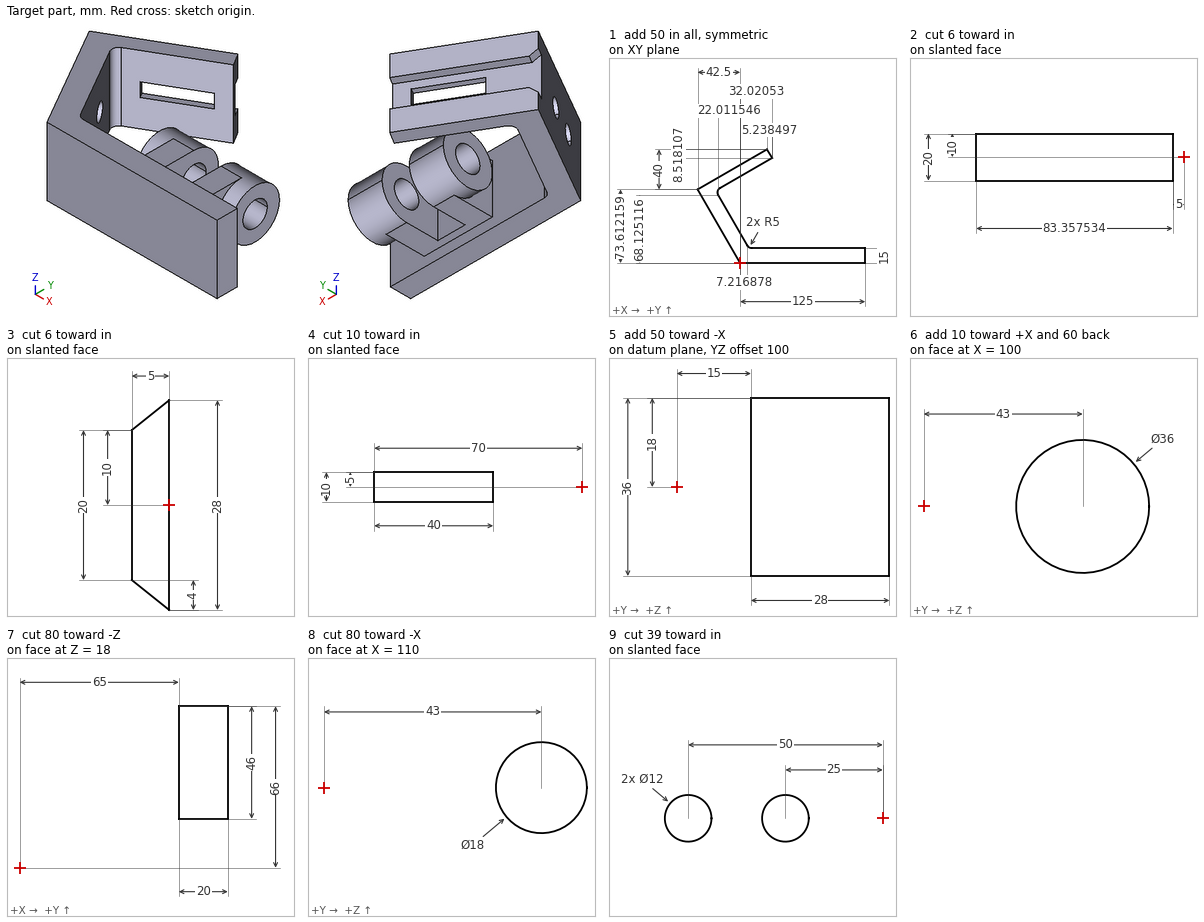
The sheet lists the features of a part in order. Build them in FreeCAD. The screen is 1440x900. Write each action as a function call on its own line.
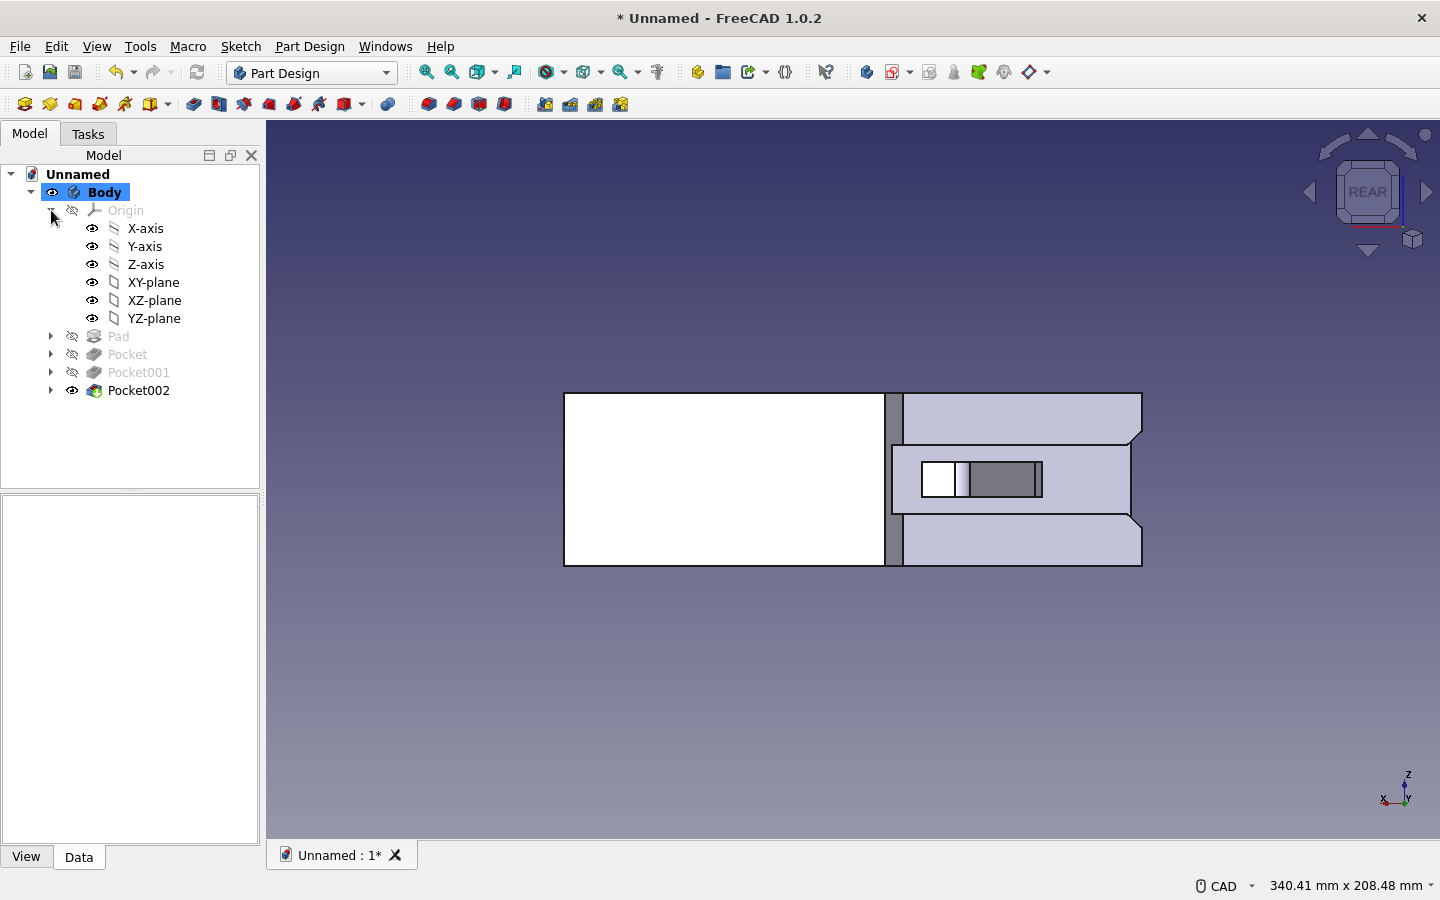
click(137, 318)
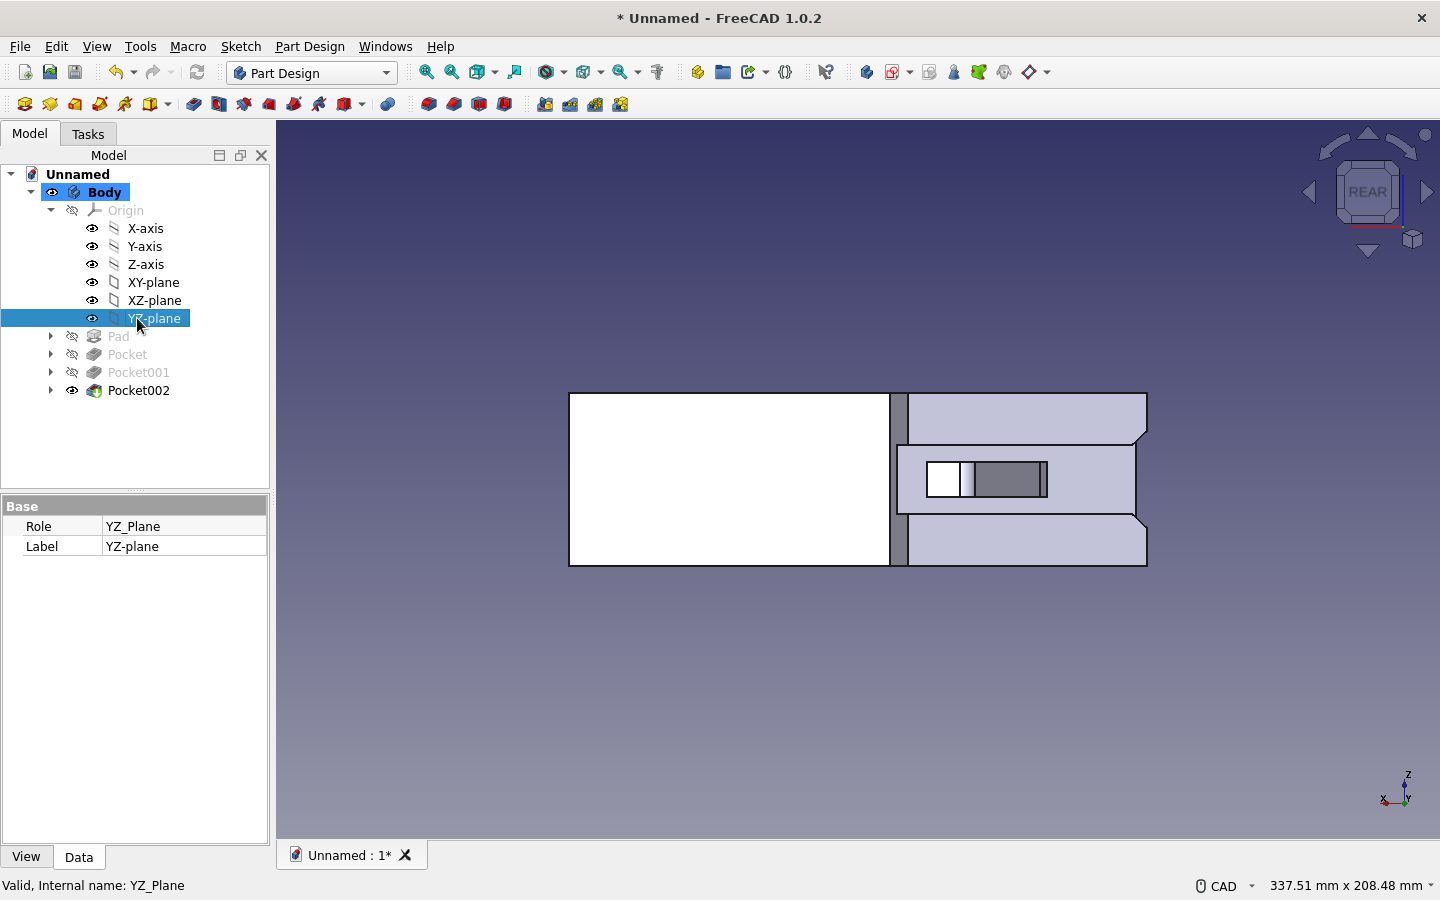
click(1028, 72)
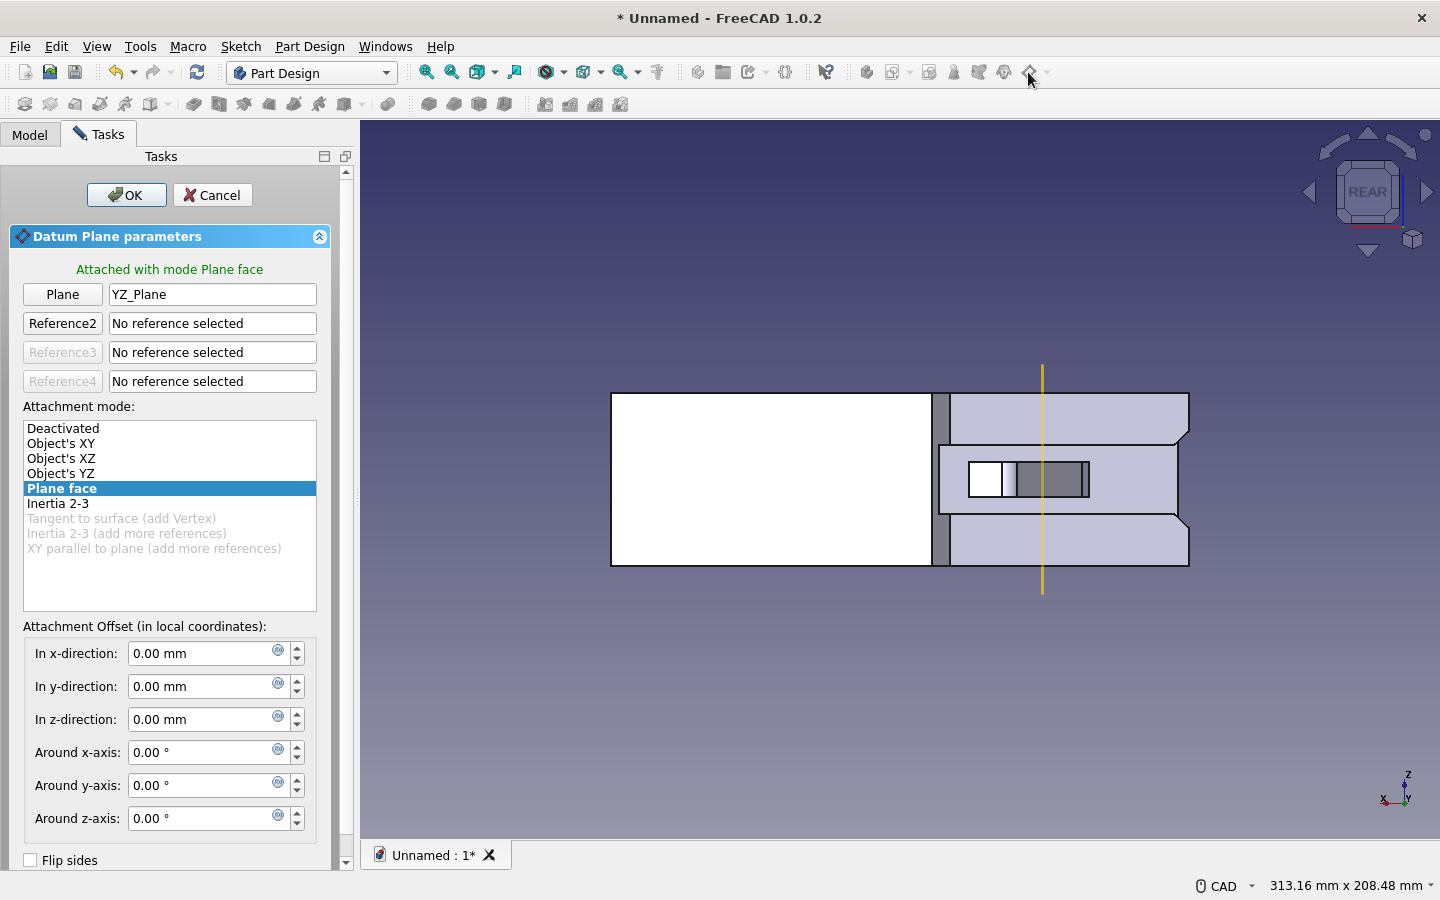
triple_click(210, 720)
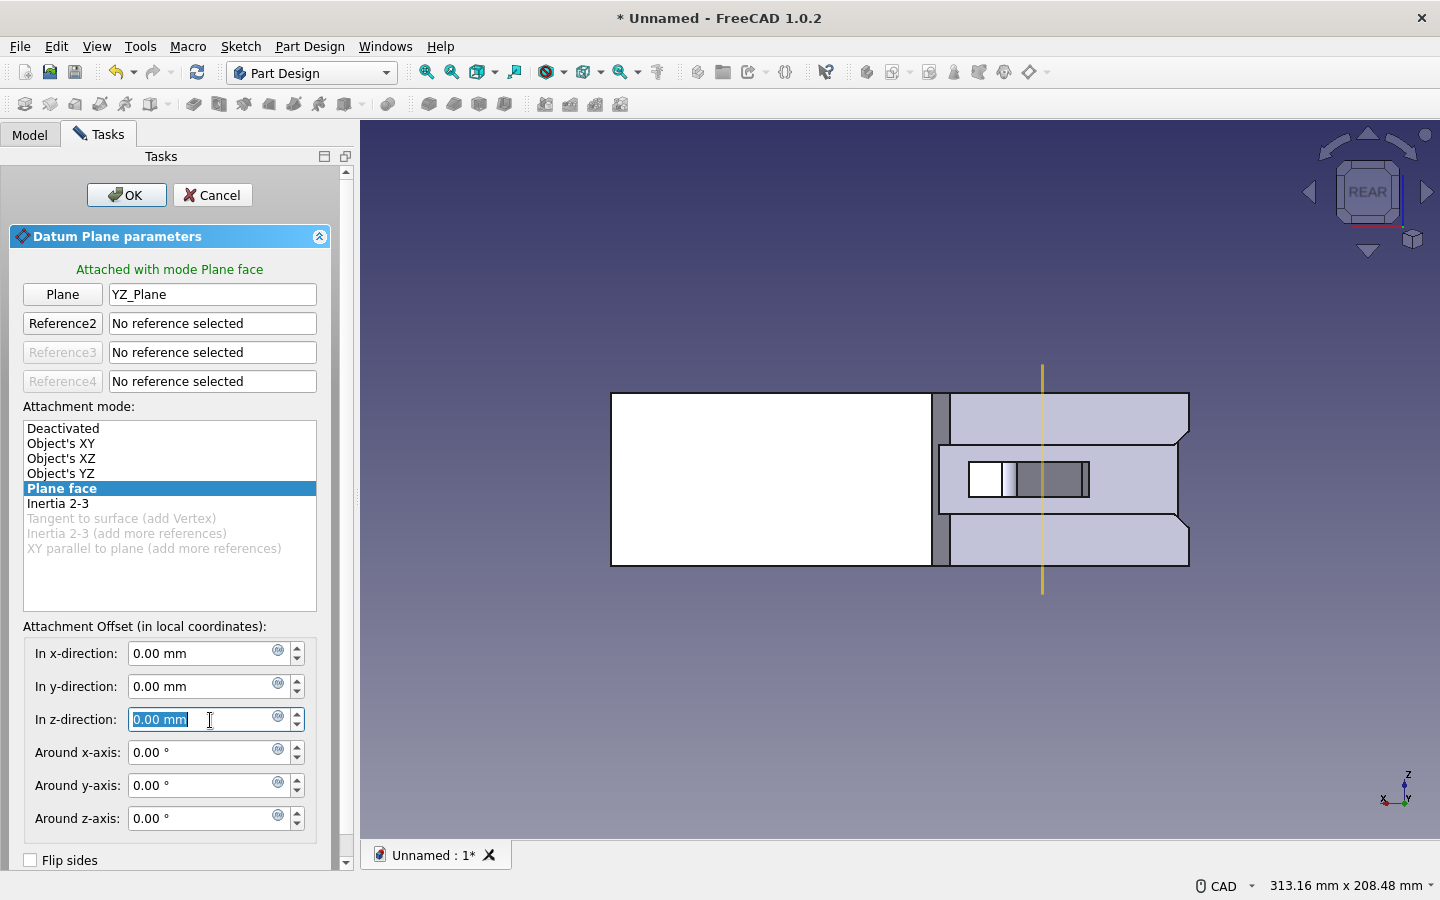
text(100)
key(Tab)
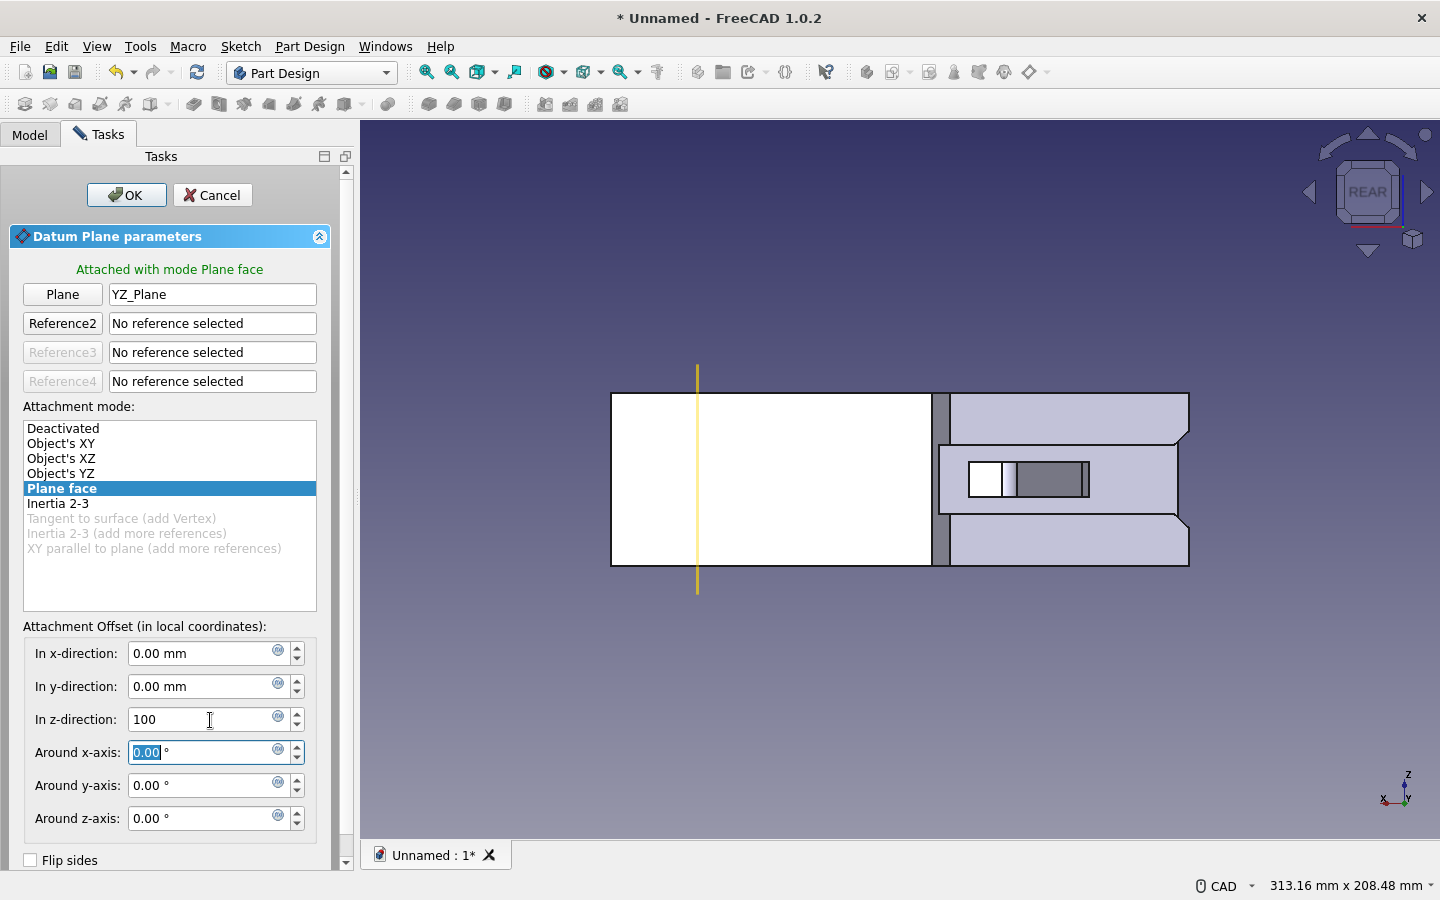
click(127, 195)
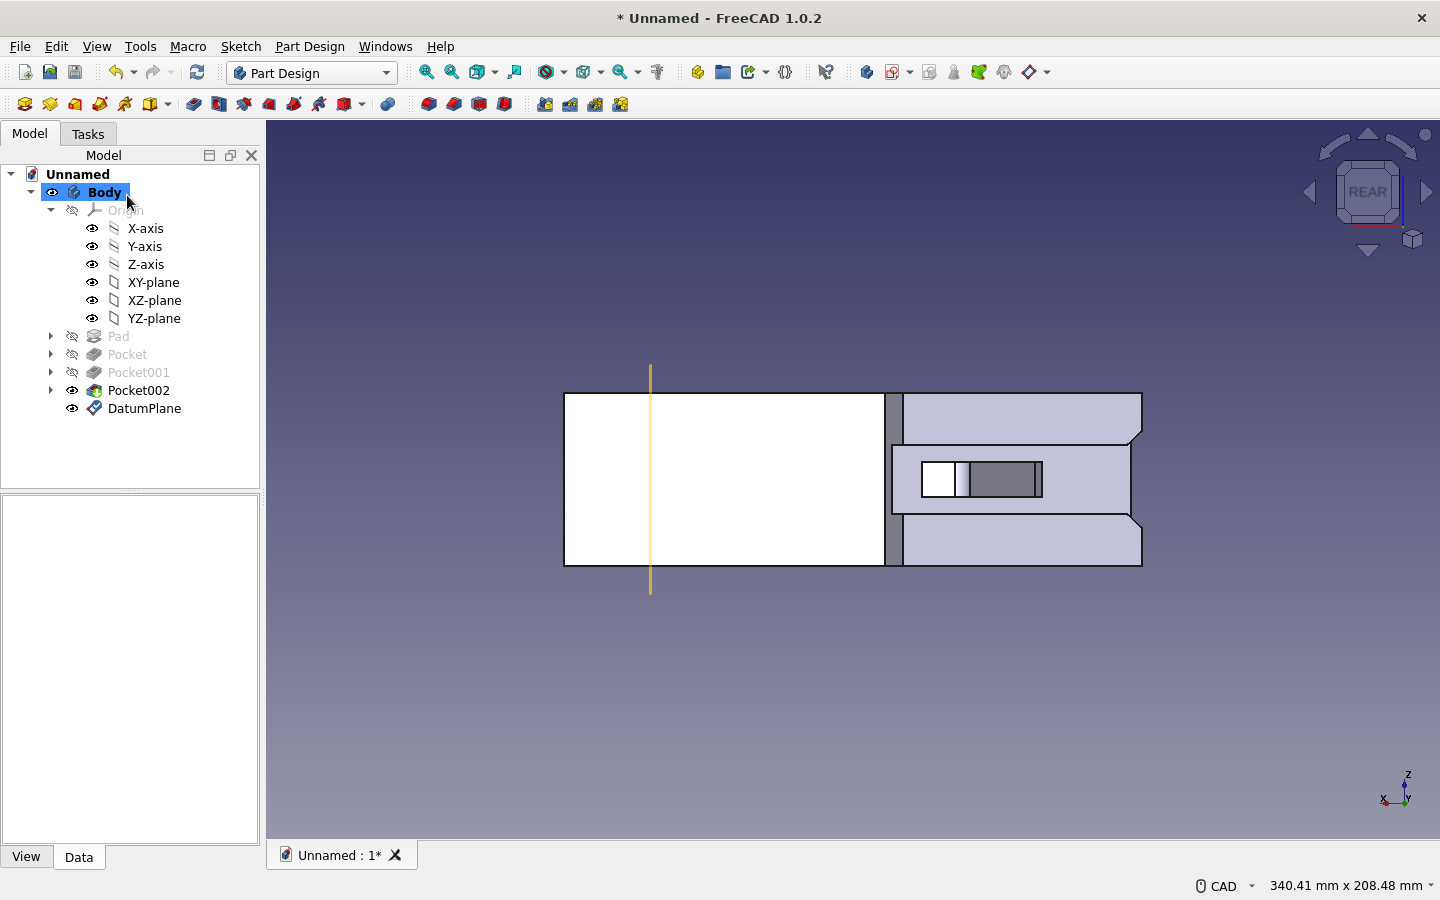
click(117, 408)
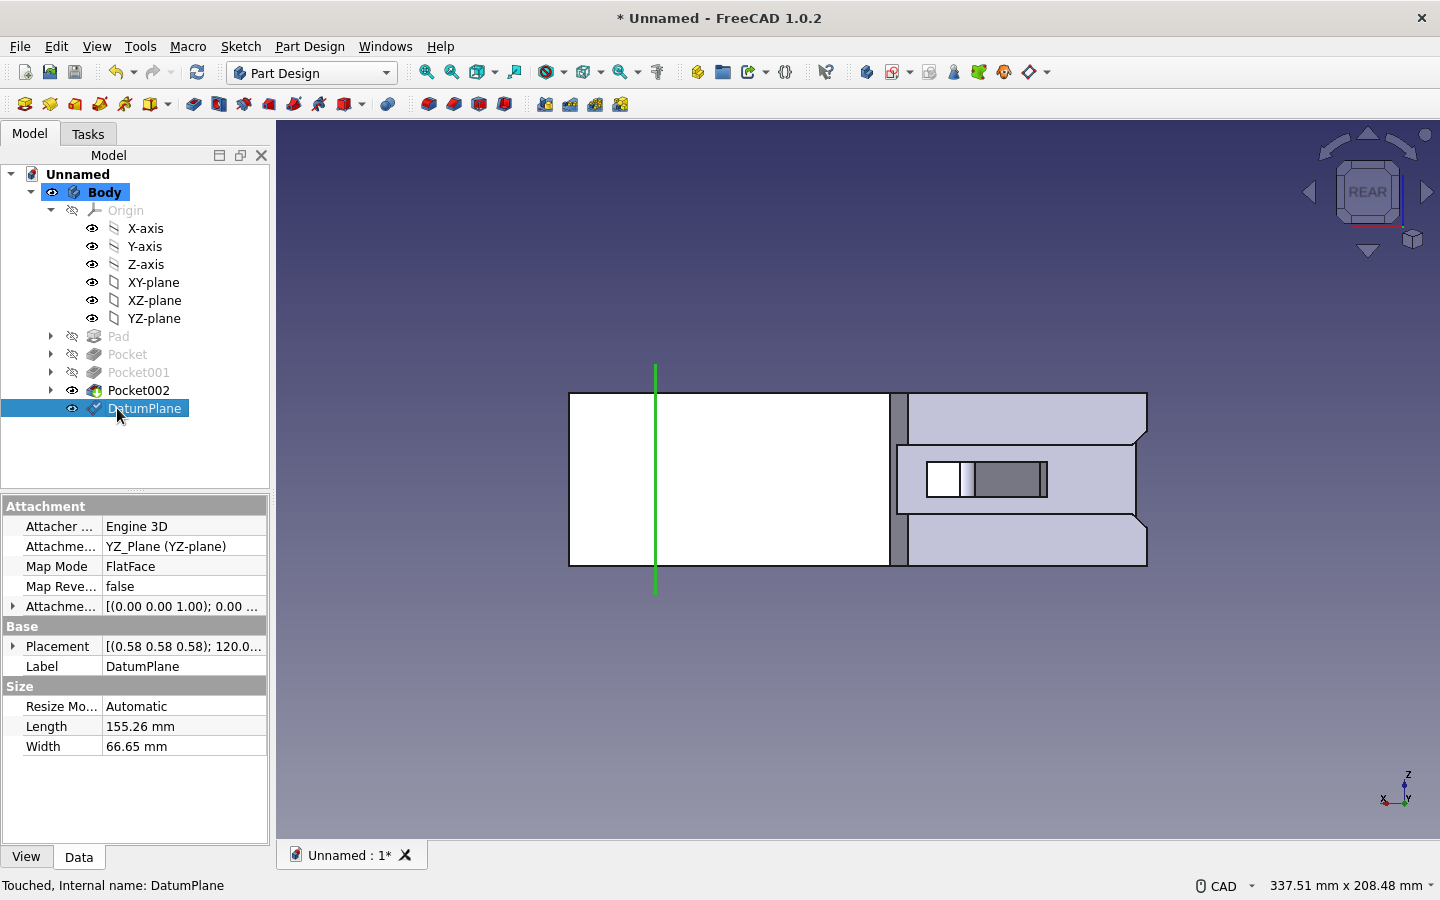
click(892, 72)